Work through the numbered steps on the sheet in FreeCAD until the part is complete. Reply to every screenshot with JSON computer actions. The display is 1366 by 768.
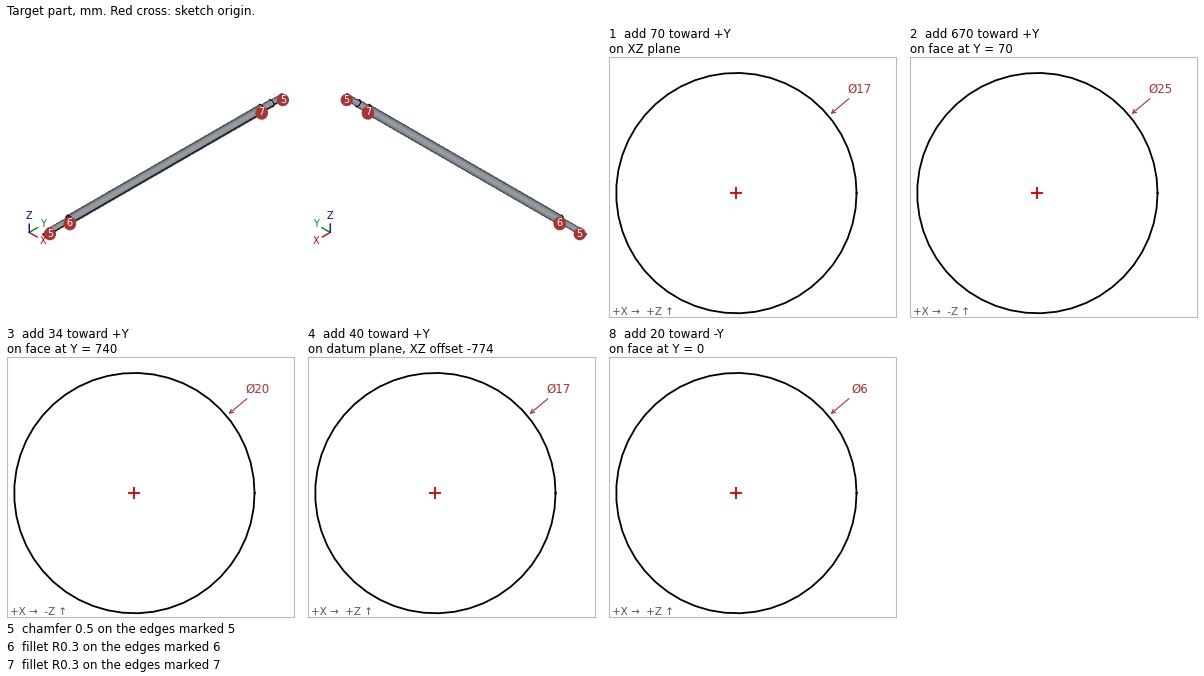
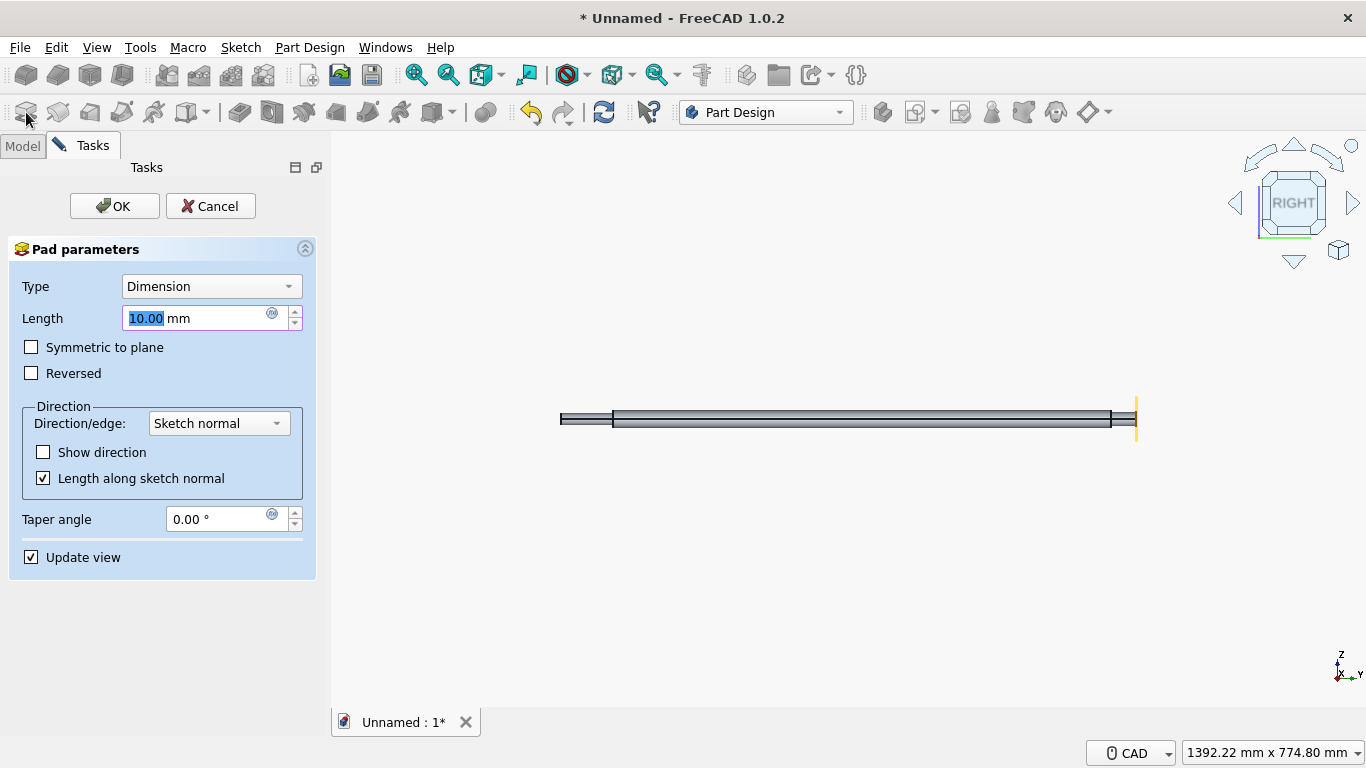
{"action": "type", "text": "40"}
{"action": "key", "text": "Tab"}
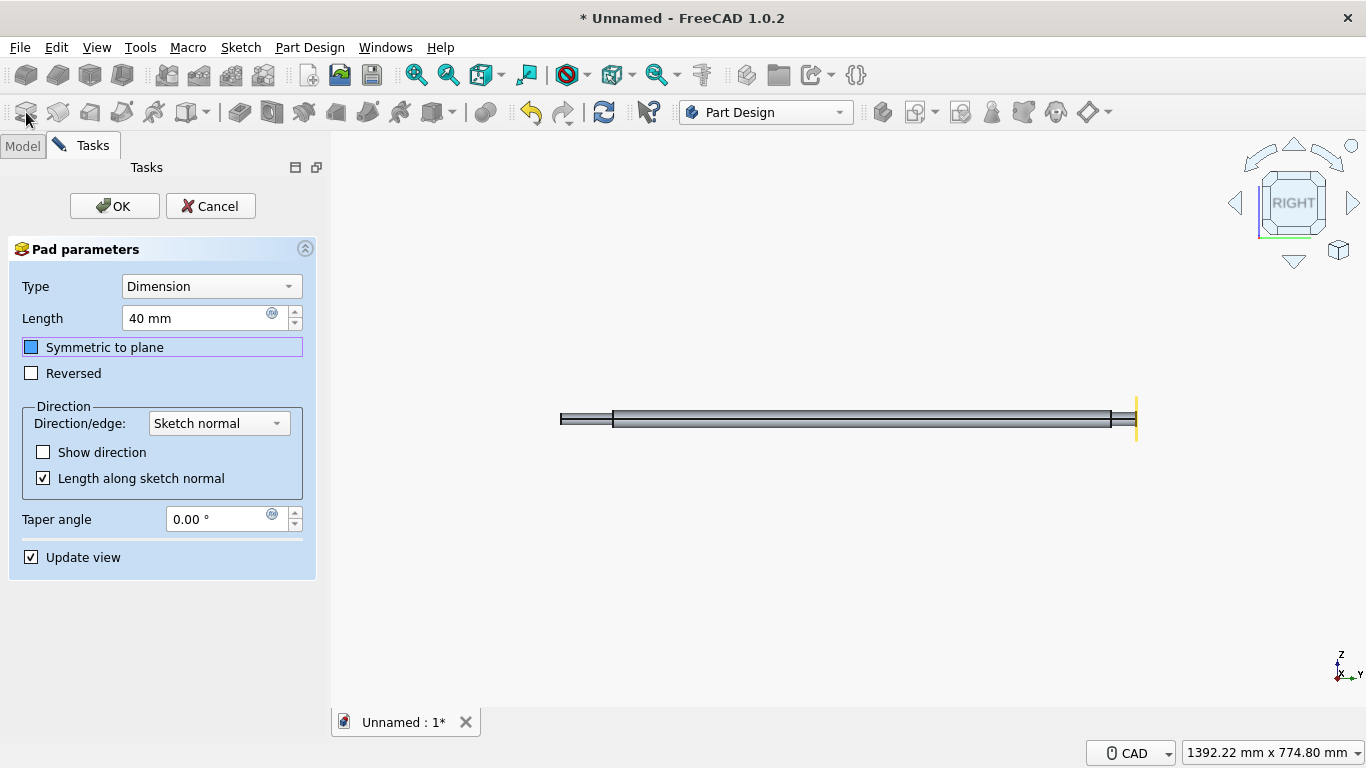
{"action": "left_click", "coordinate": [30, 373]}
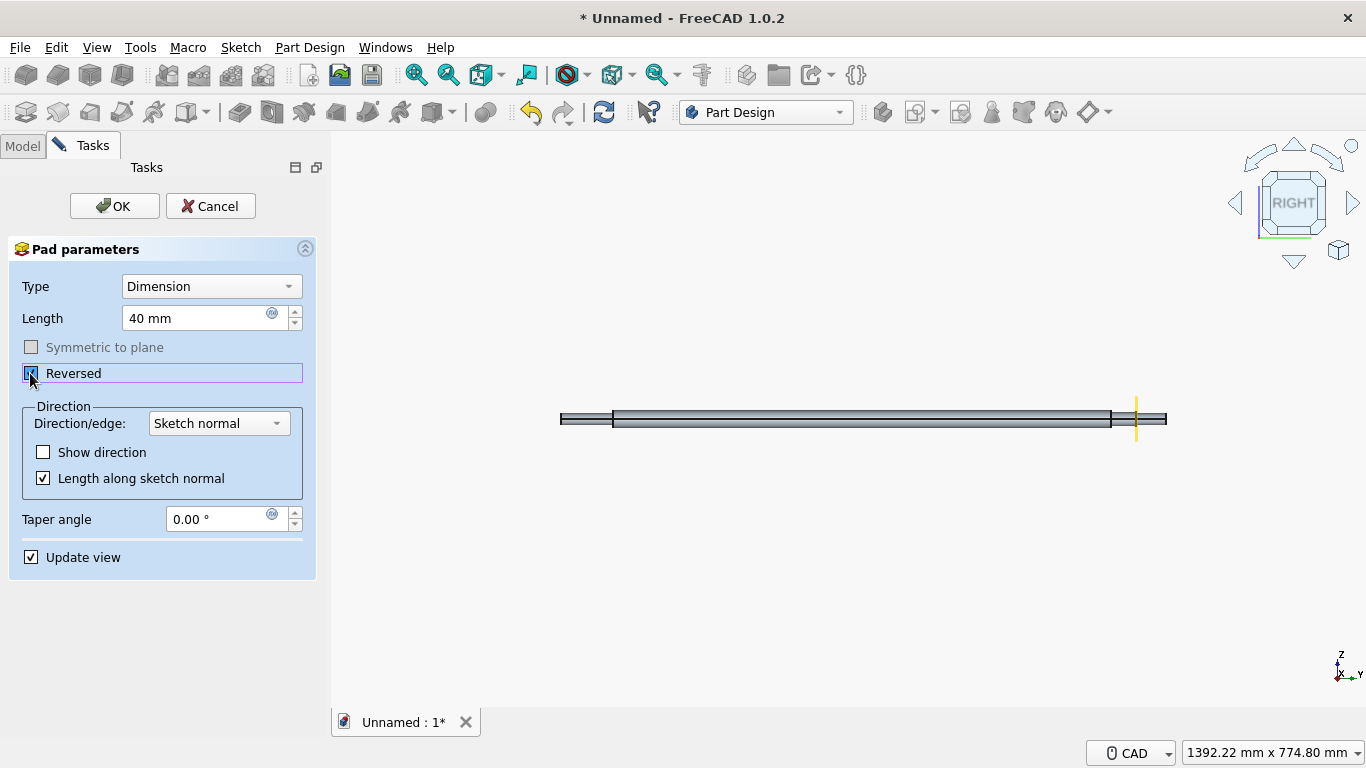
{"action": "left_click", "coordinate": [115, 206]}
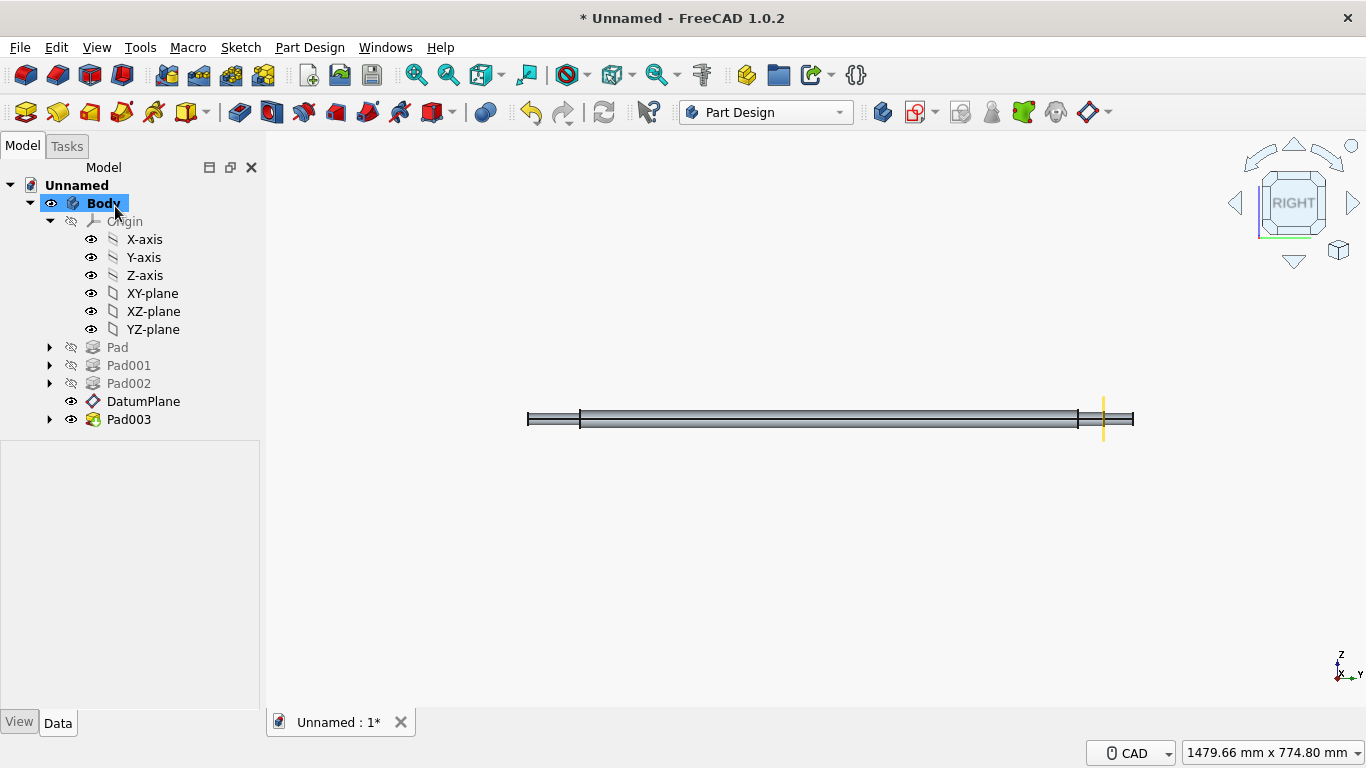
{"action": "left_click", "coordinate": [116, 401]}
{"action": "key", "text": "space"}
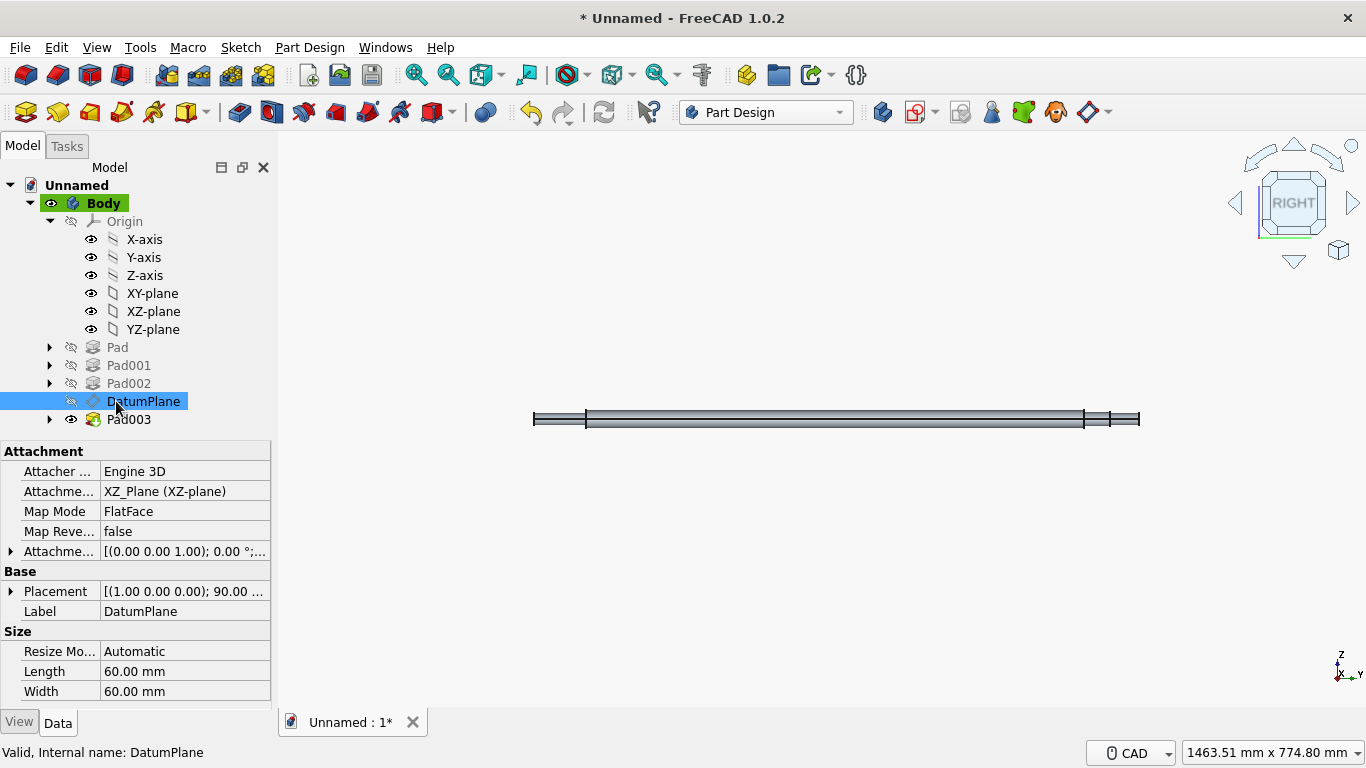
{"action": "left_click", "coordinate": [1139, 412]}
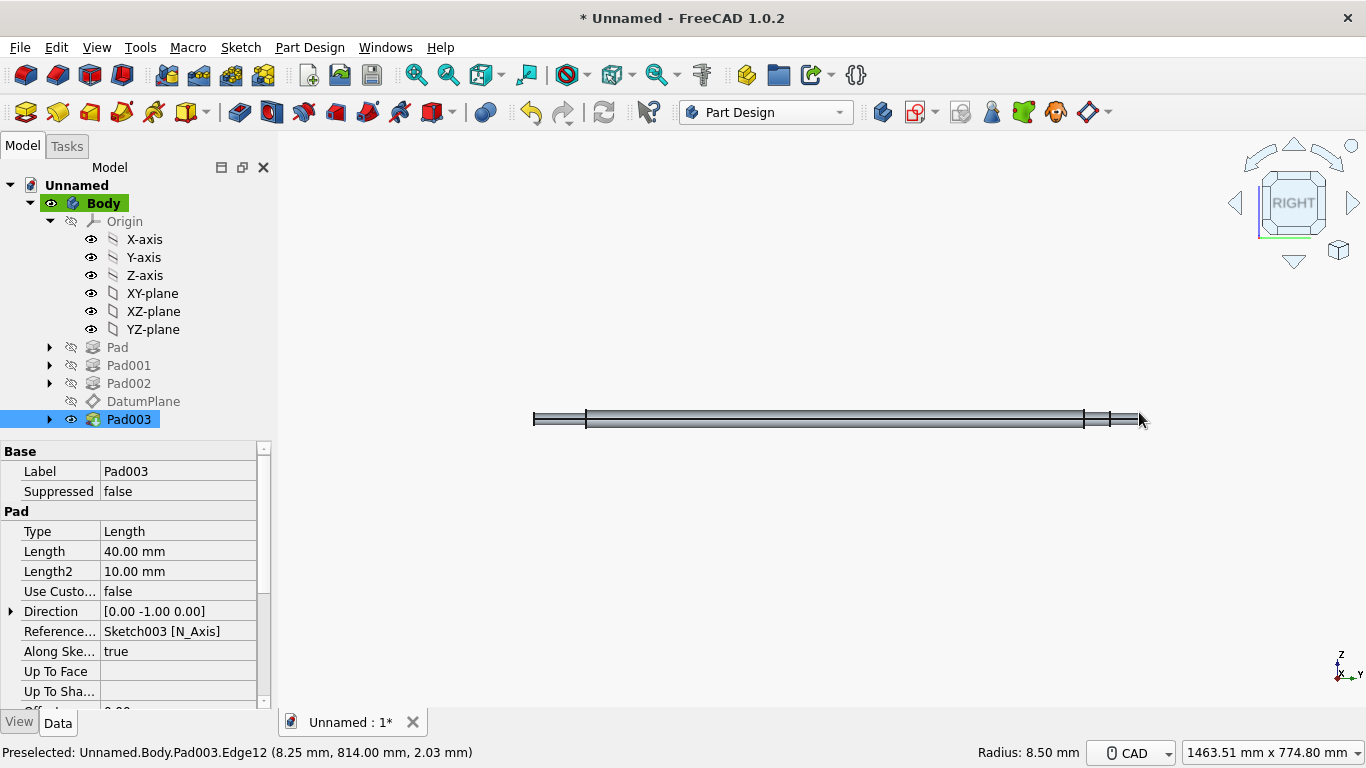
{"action": "left_click", "coordinate": [534, 412], "text": "ctrl"}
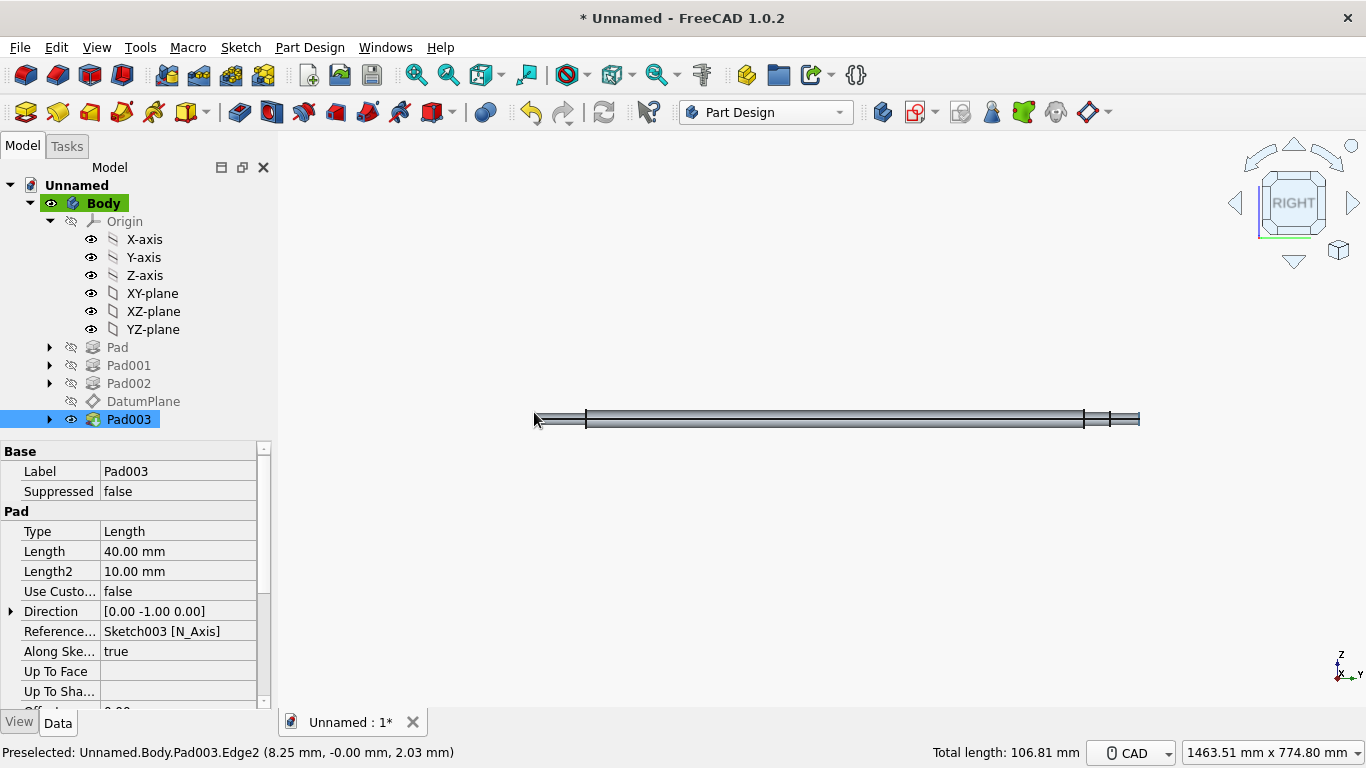
{"action": "left_click", "coordinate": [586, 427], "text": "ctrl"}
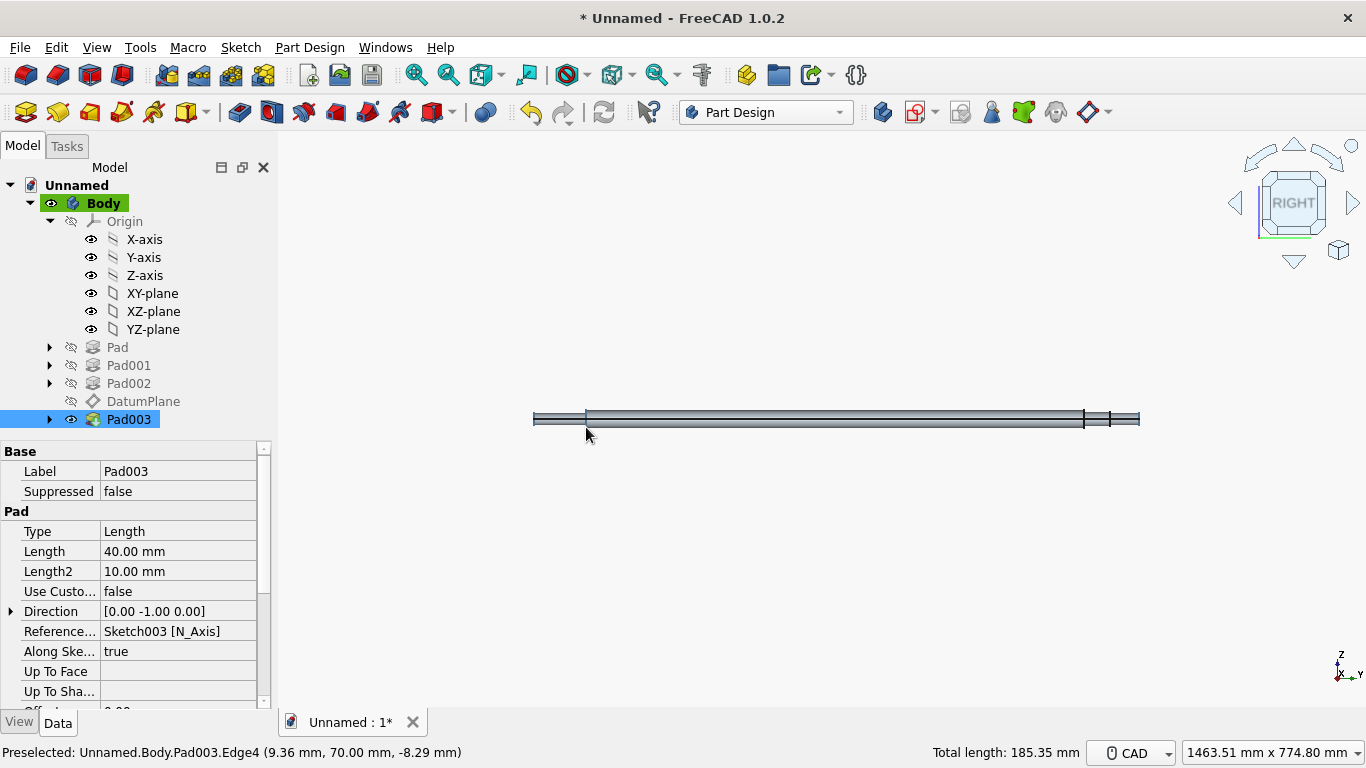
{"action": "left_click", "coordinate": [1084, 427], "text": "ctrl"}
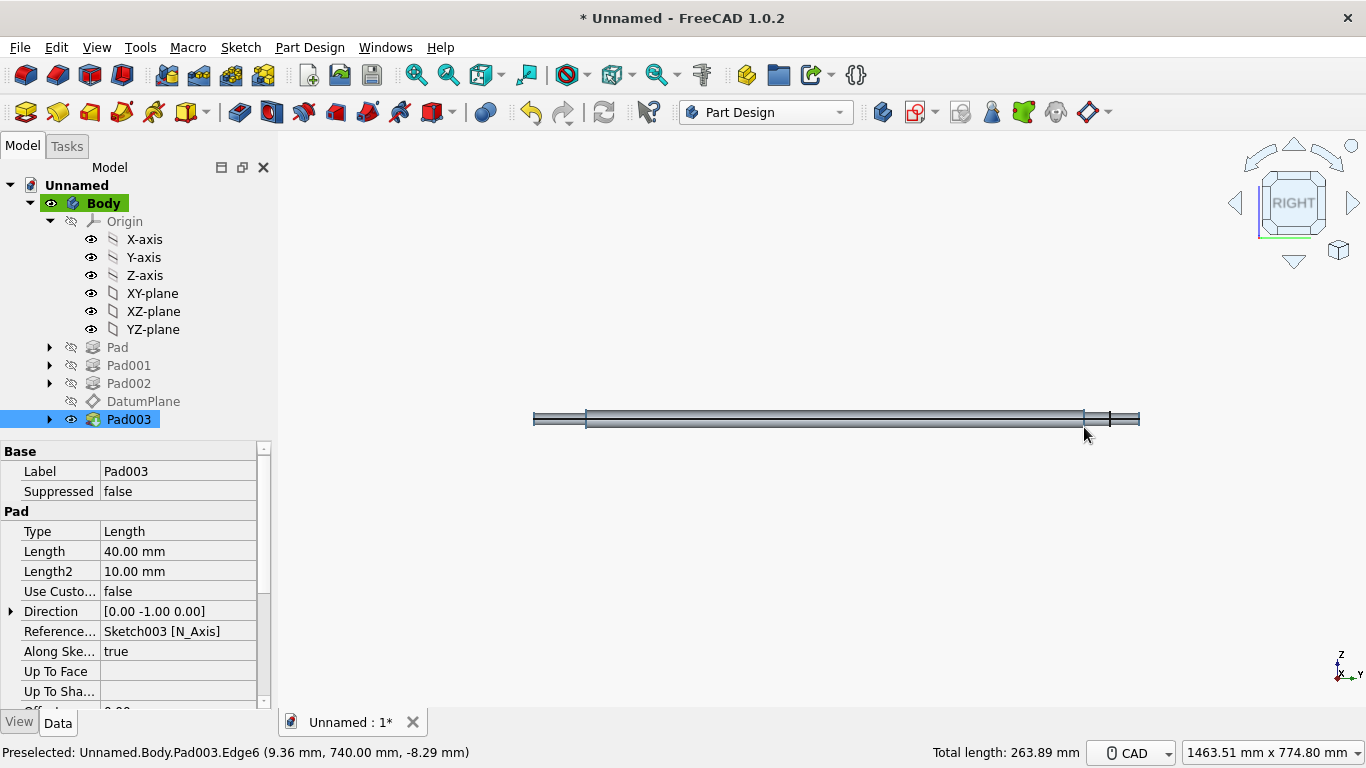
{"action": "left_click", "coordinate": [58, 76]}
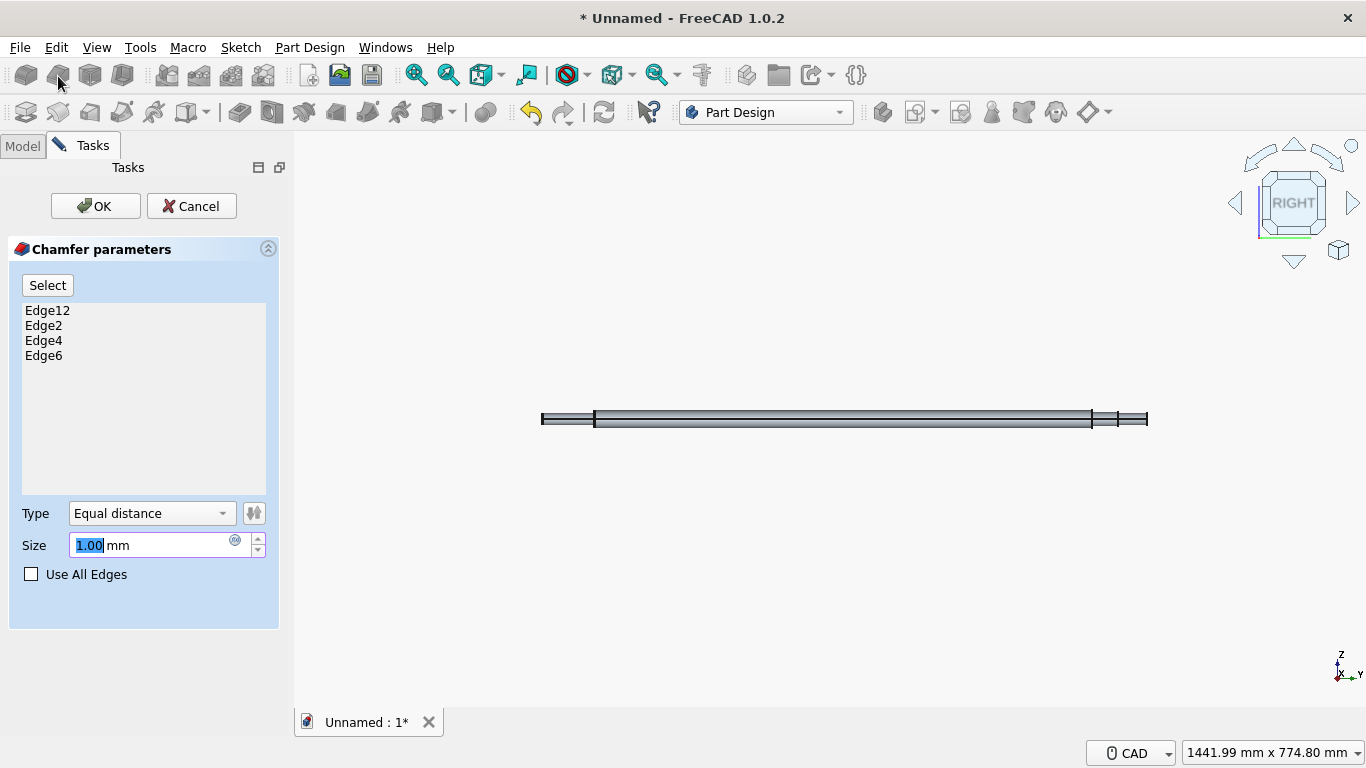
{"action": "type", "text": "0.5"}
{"action": "key", "text": "Tab"}